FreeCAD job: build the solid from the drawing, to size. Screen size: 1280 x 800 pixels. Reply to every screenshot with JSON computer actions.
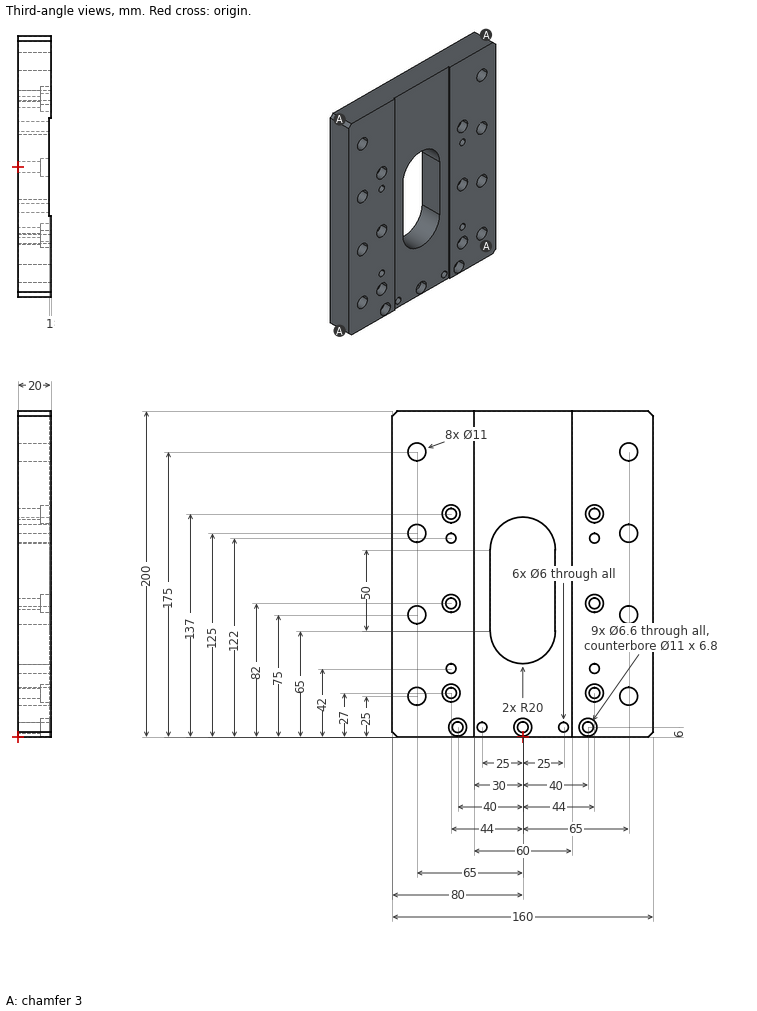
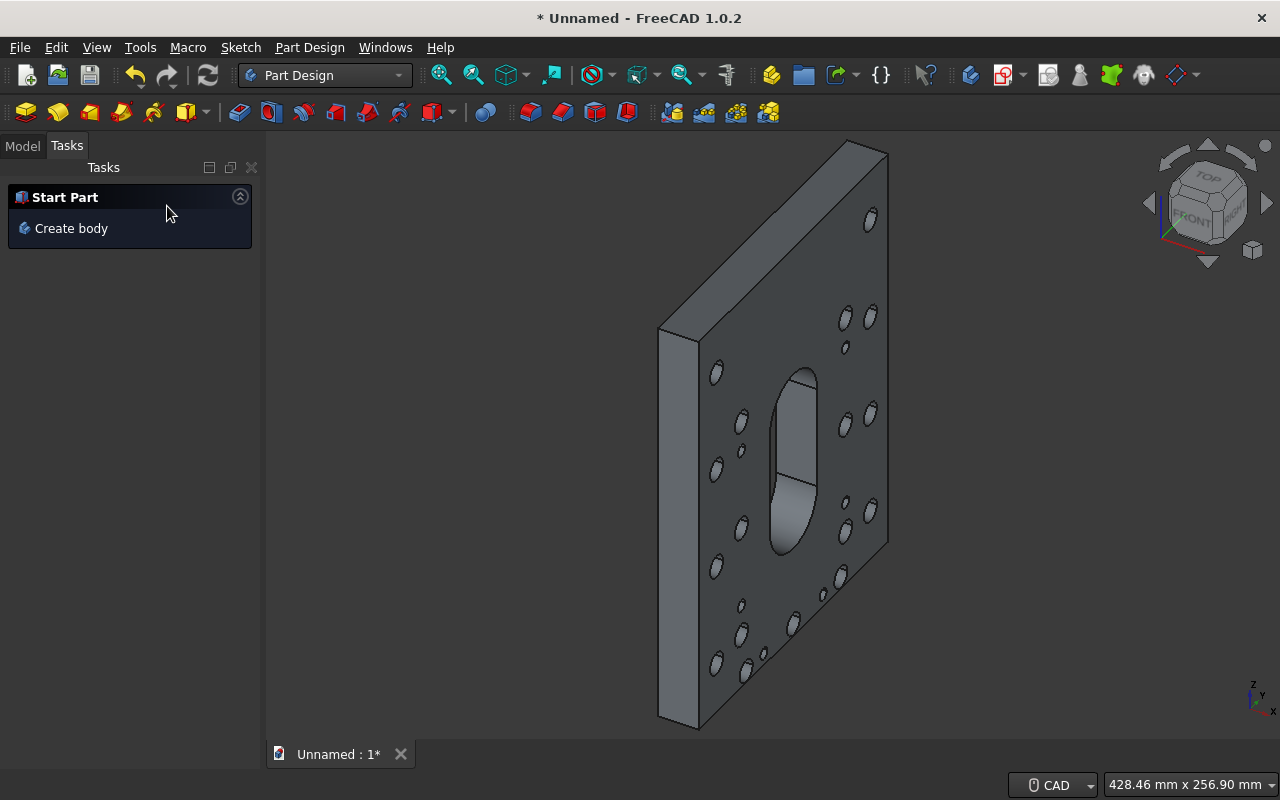
{"action": "left_click", "coordinate": [766, 357]}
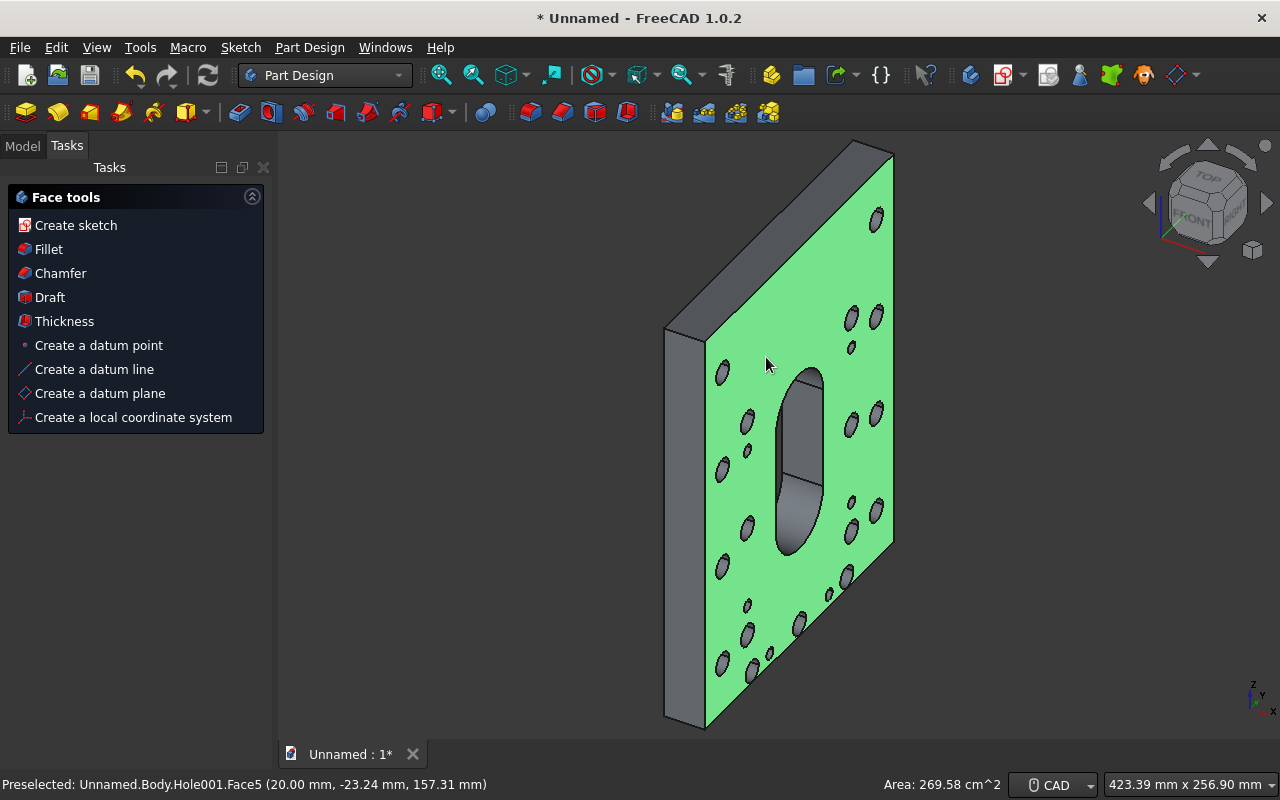
{"action": "left_click", "coordinate": [1004, 76]}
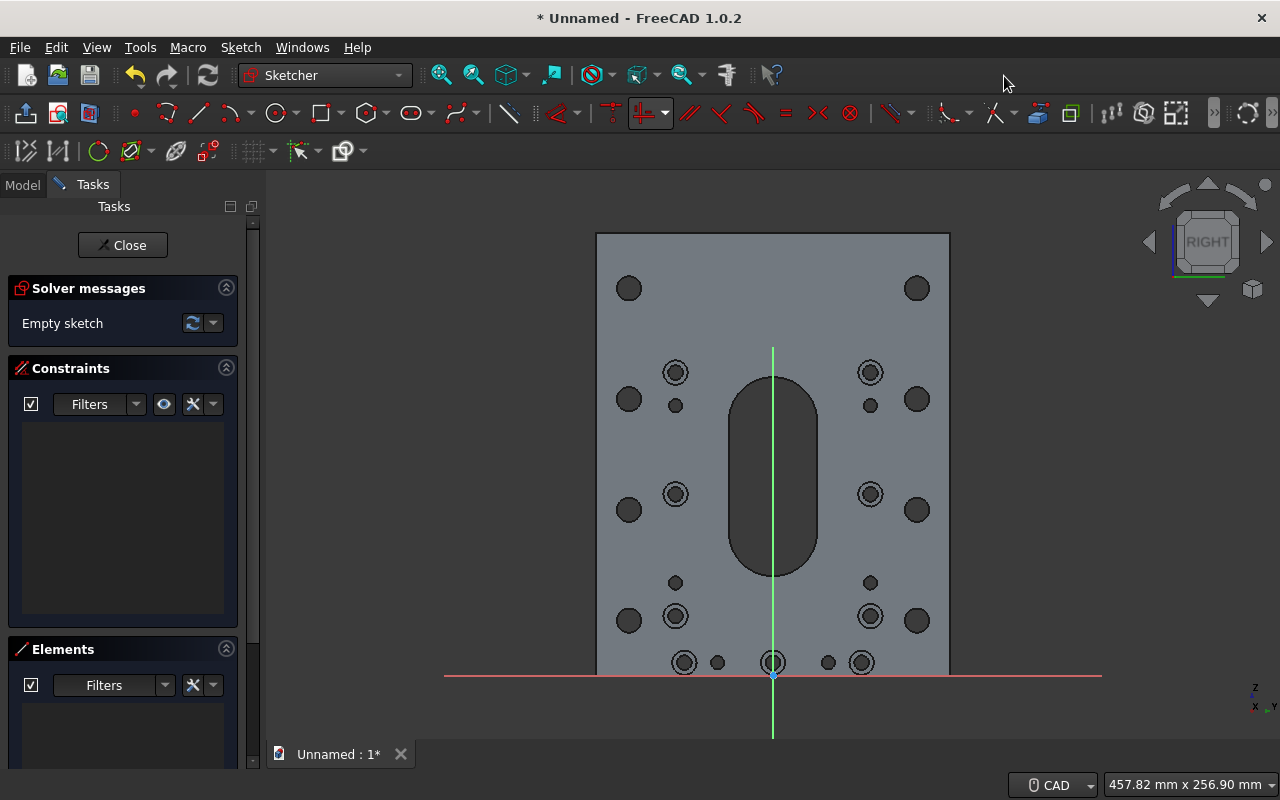
{"action": "key", "text": "g r"}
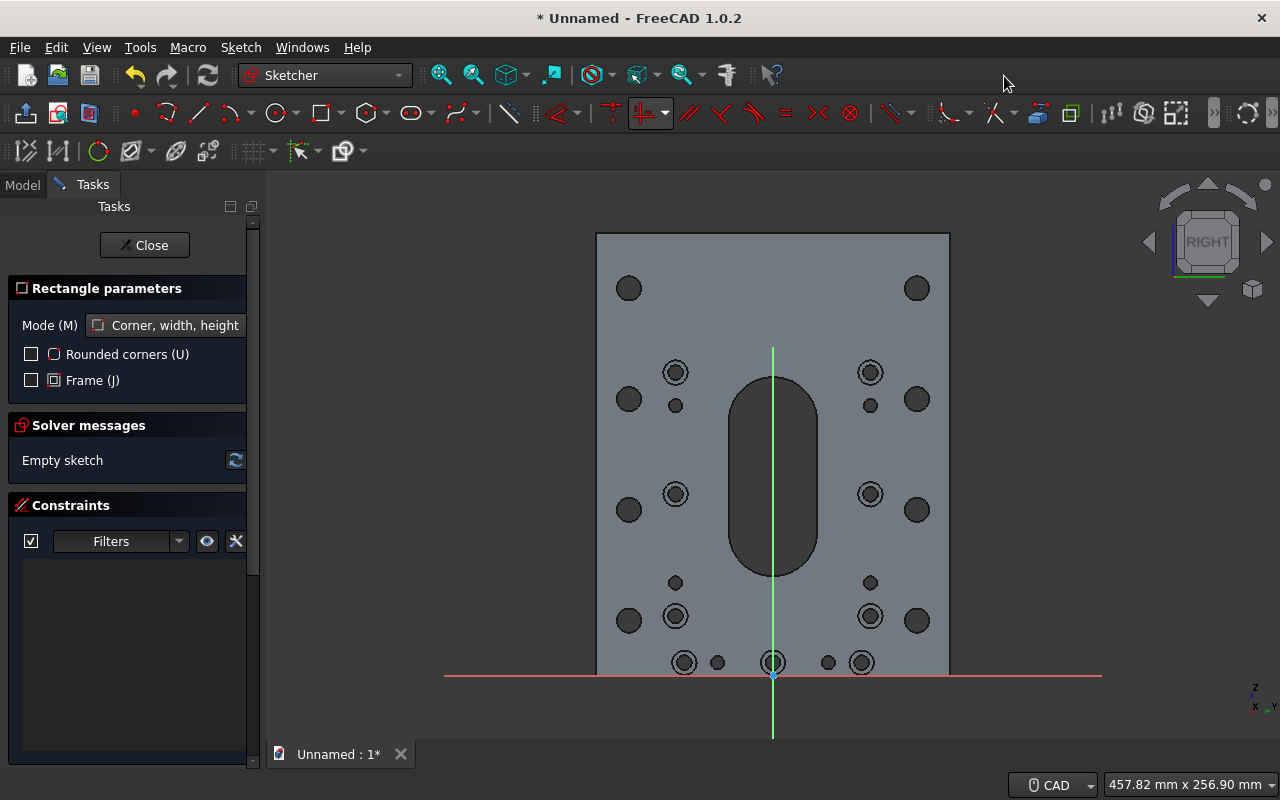
{"action": "left_click", "coordinate": [707, 233]}
{"action": "left_click", "coordinate": [839, 676]}
{"action": "key", "text": "Escape"}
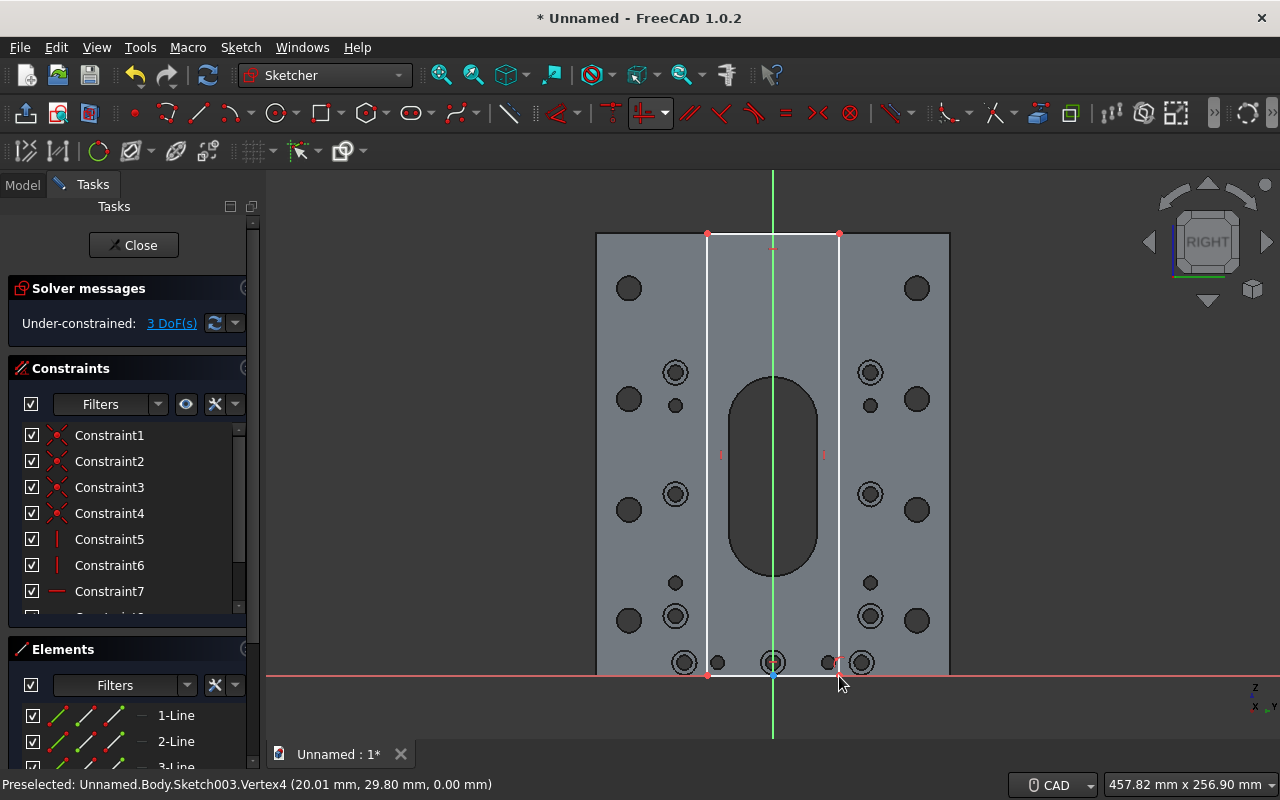
{"action": "key", "text": "d"}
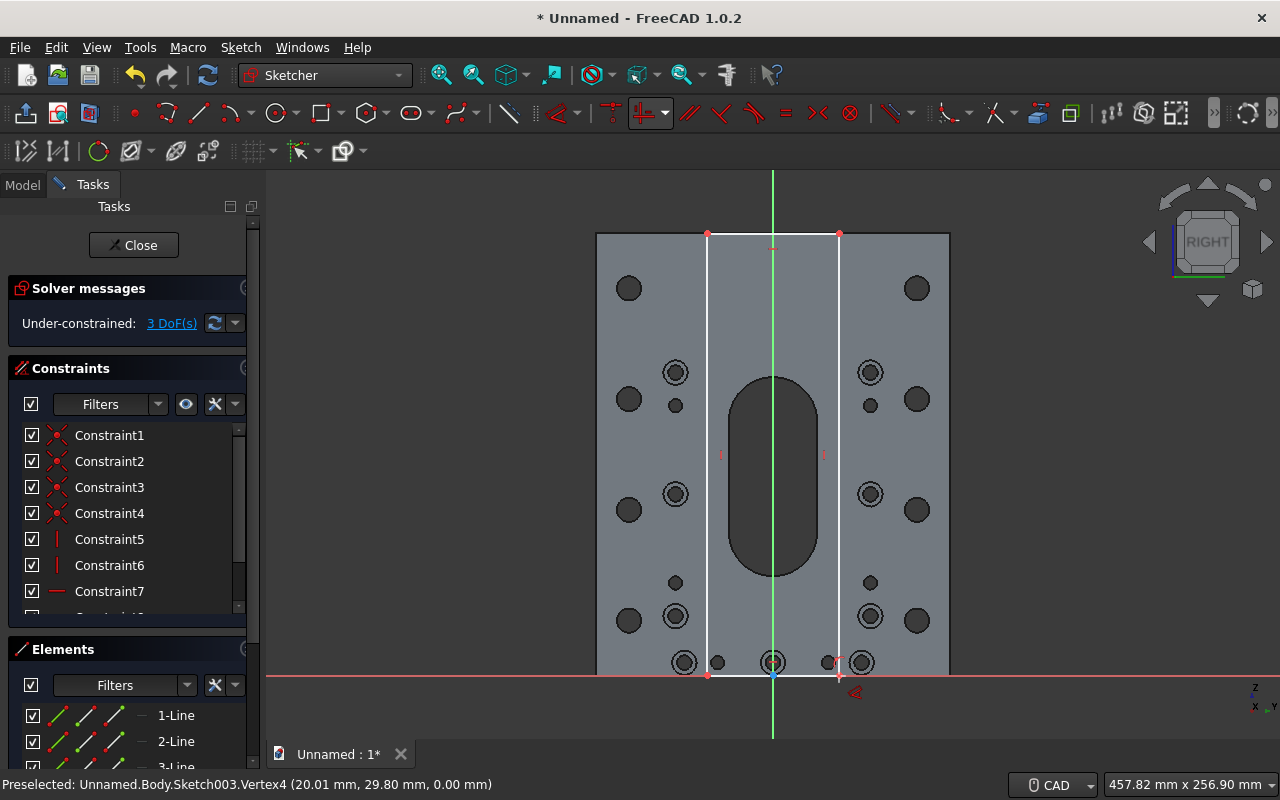
{"action": "left_click", "coordinate": [747, 676]}
{"action": "left_click", "coordinate": [743, 710]}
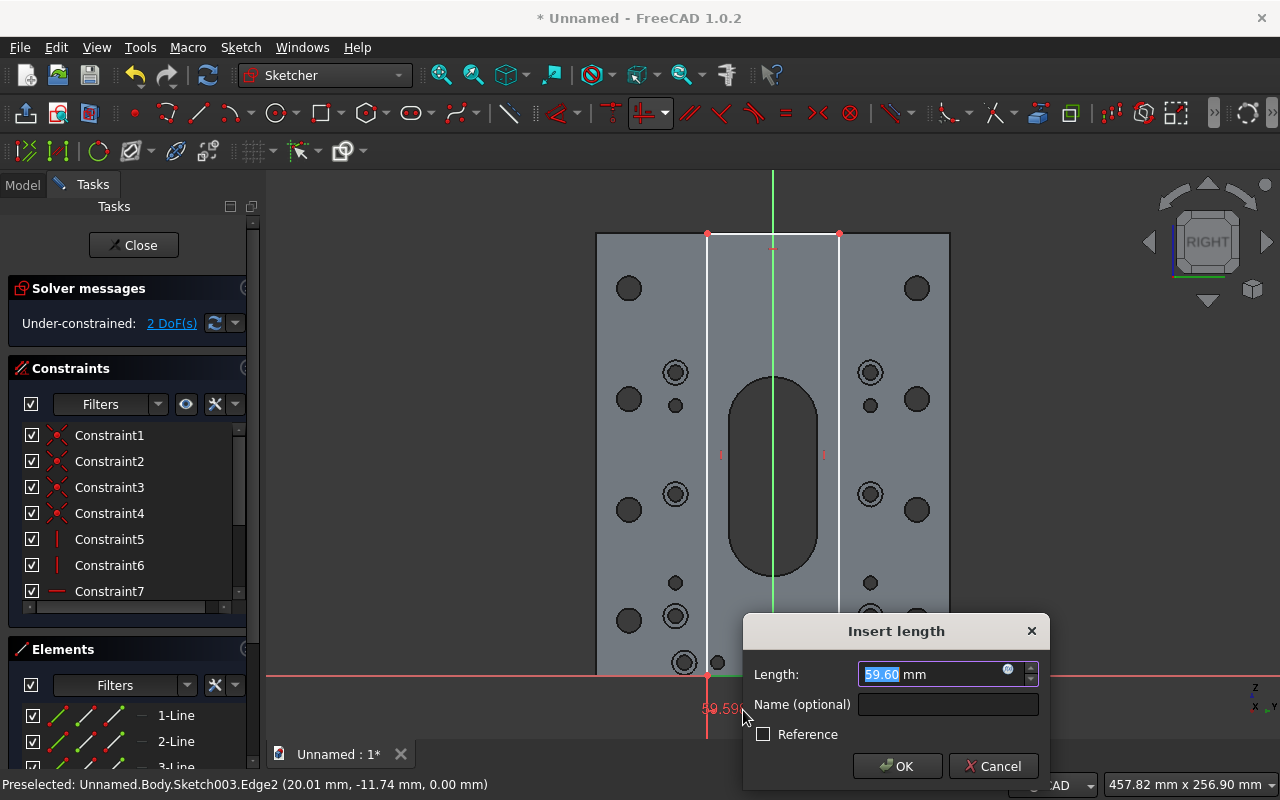
{"action": "type", "text": "60"}
{"action": "key", "text": "Return"}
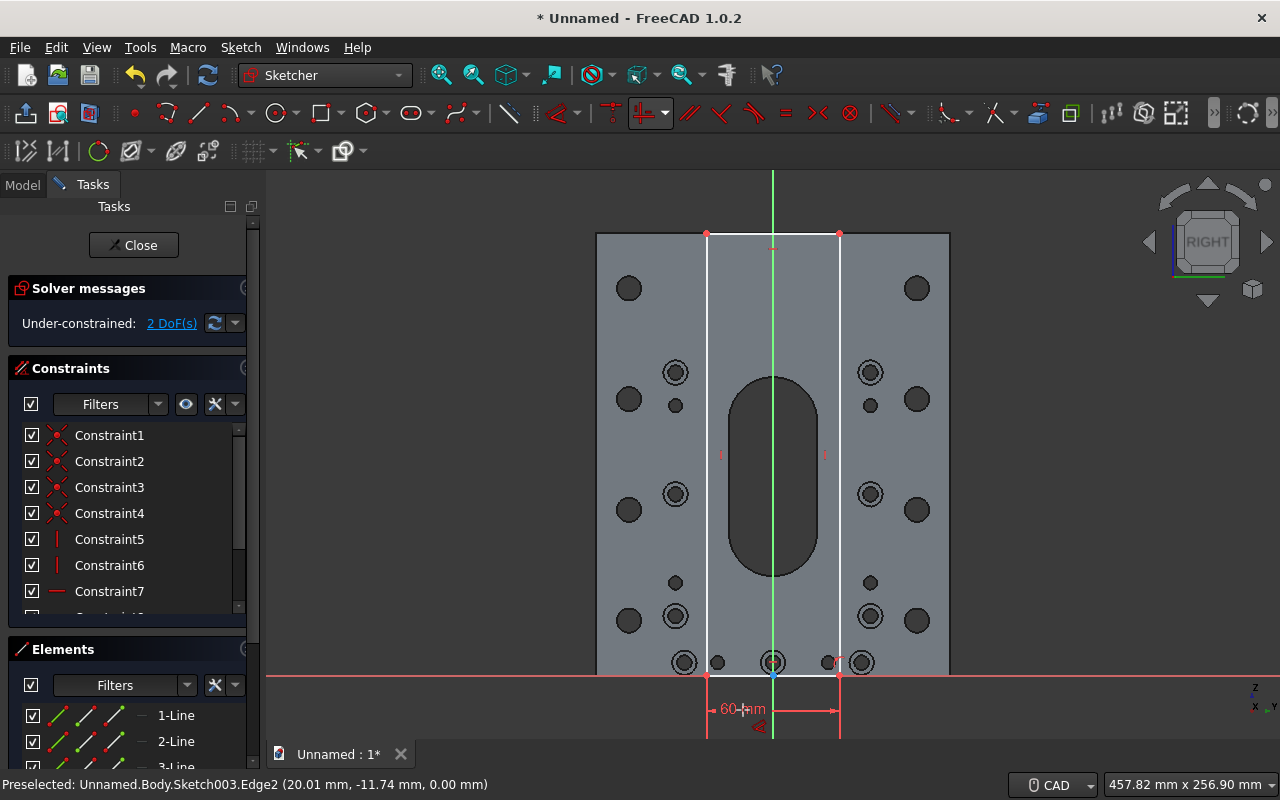
{"action": "left_click", "coordinate": [707, 367]}
{"action": "left_click", "coordinate": [673, 455]}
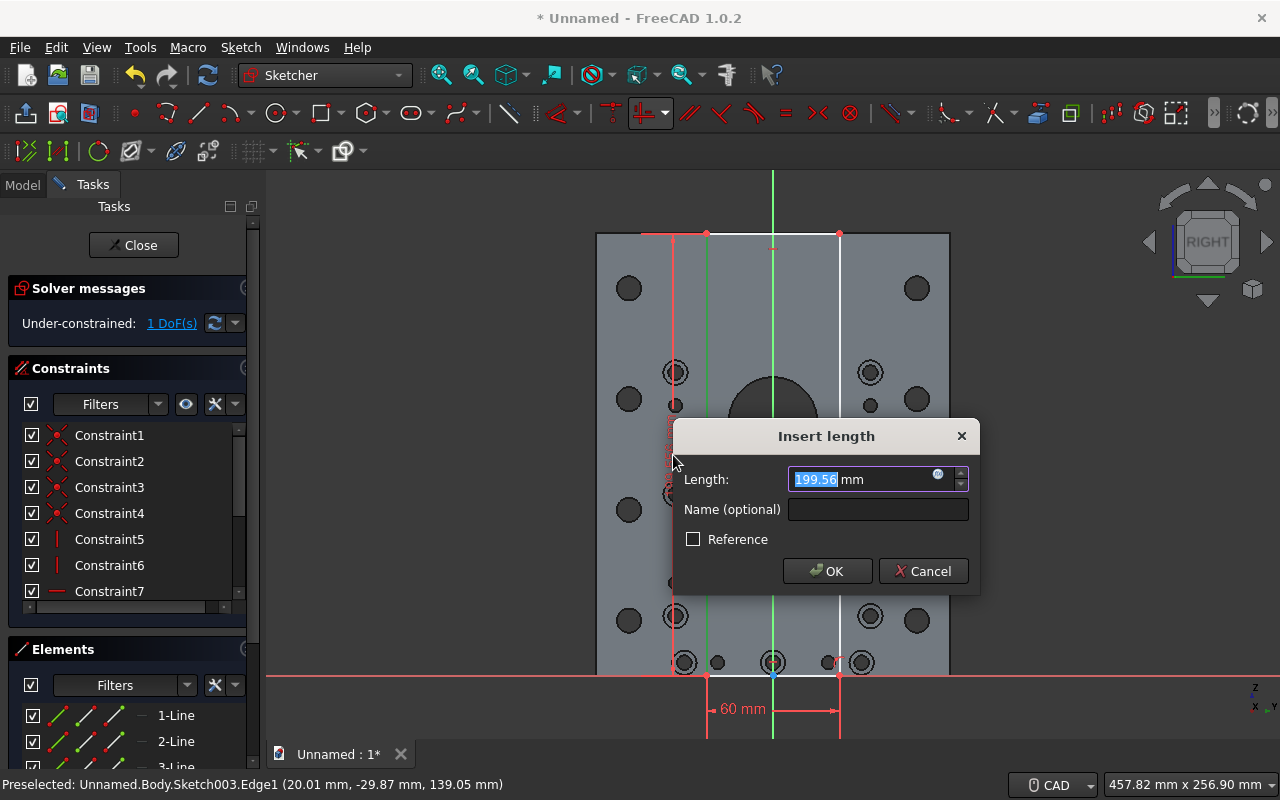
{"action": "type", "text": "200"}
{"action": "key", "text": "Return"}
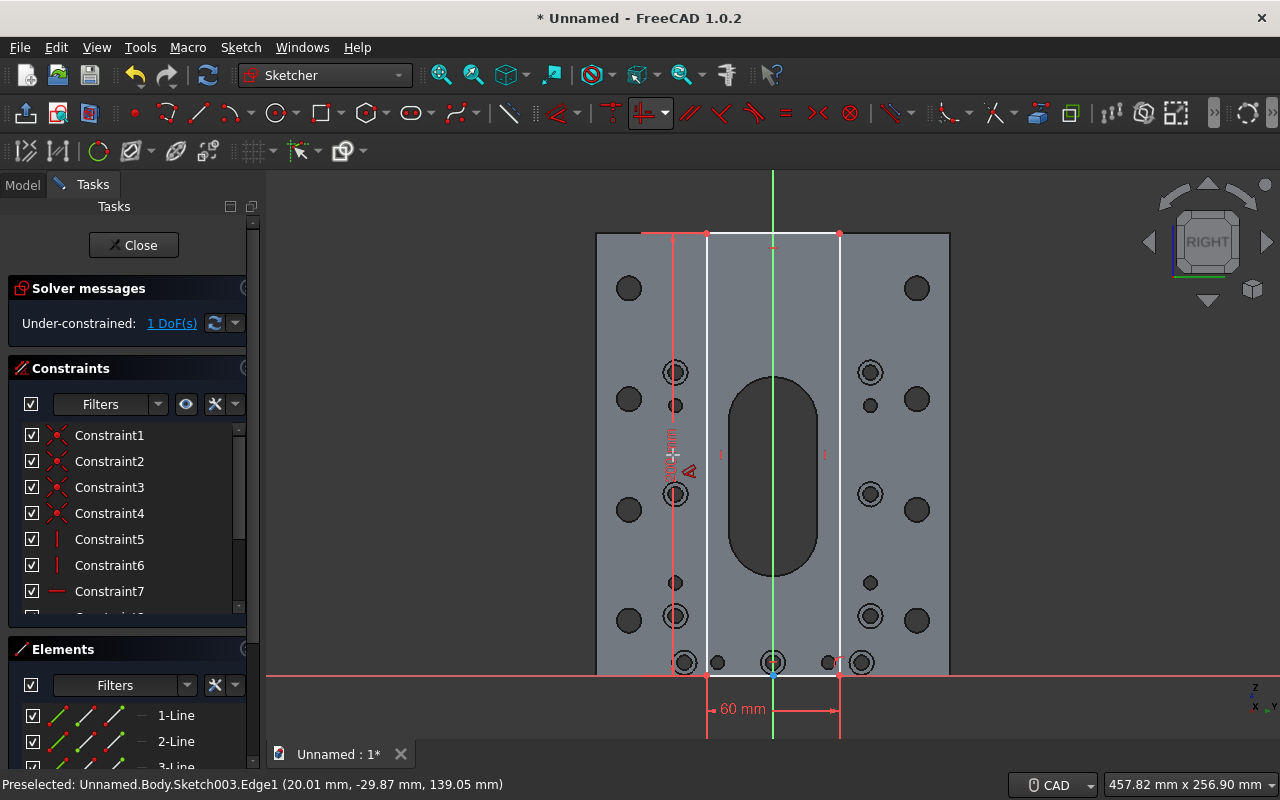
{"action": "left_click", "coordinate": [707, 233]}
{"action": "left_click", "coordinate": [740, 199]}